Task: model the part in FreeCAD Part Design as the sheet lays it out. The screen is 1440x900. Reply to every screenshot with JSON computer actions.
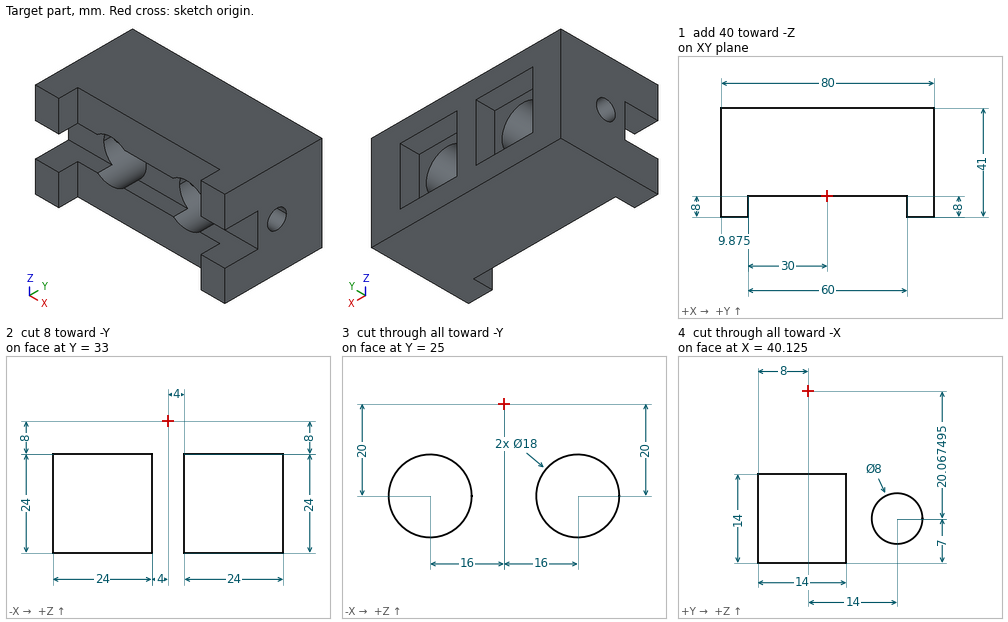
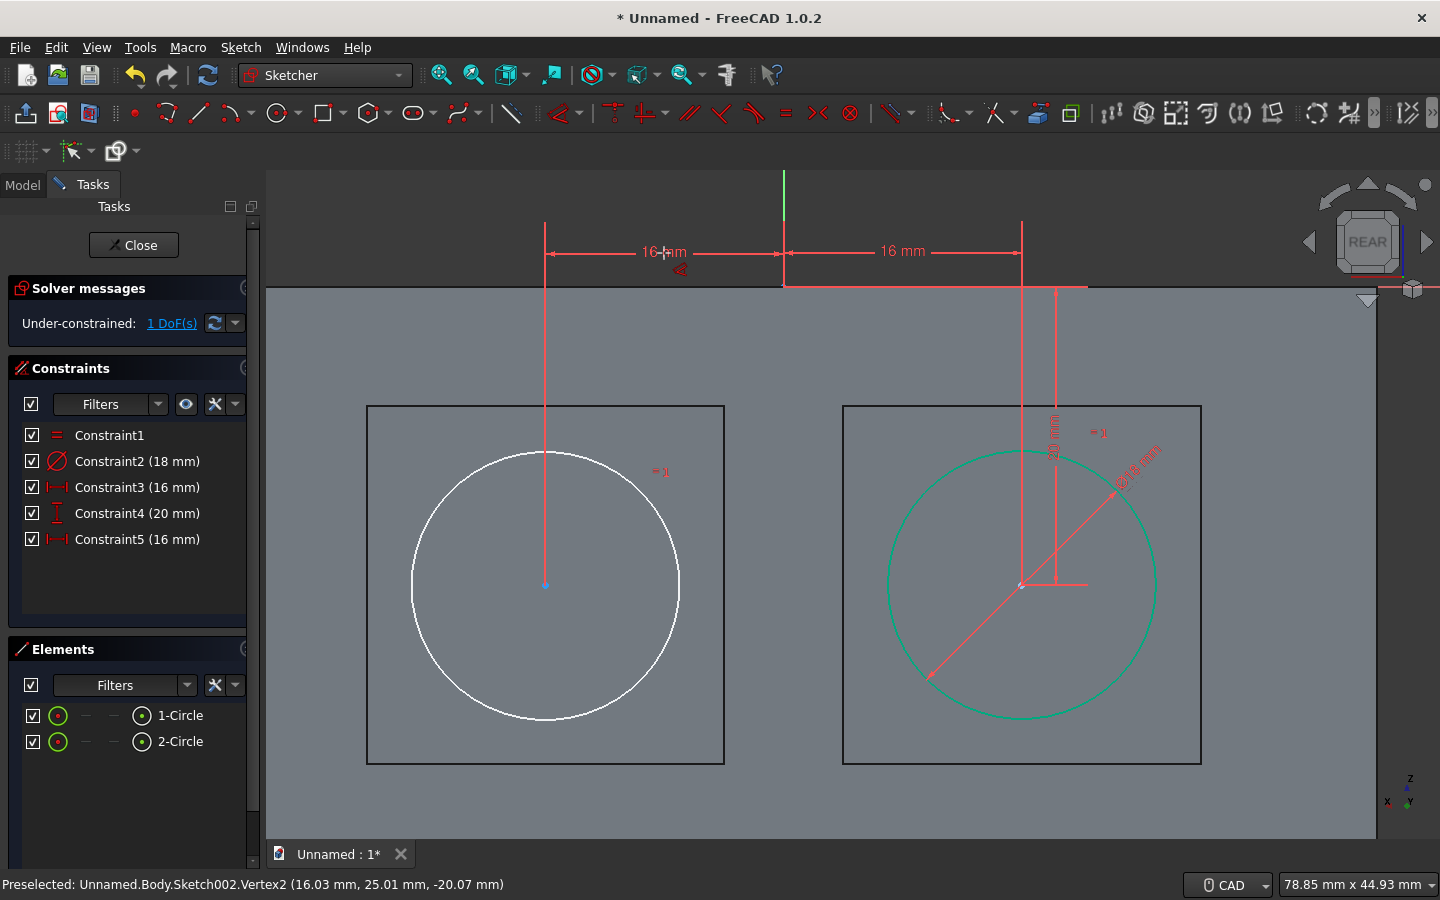
{"action": "left_click", "coordinate": [545, 586]}
{"action": "left_click", "coordinate": [511, 437]}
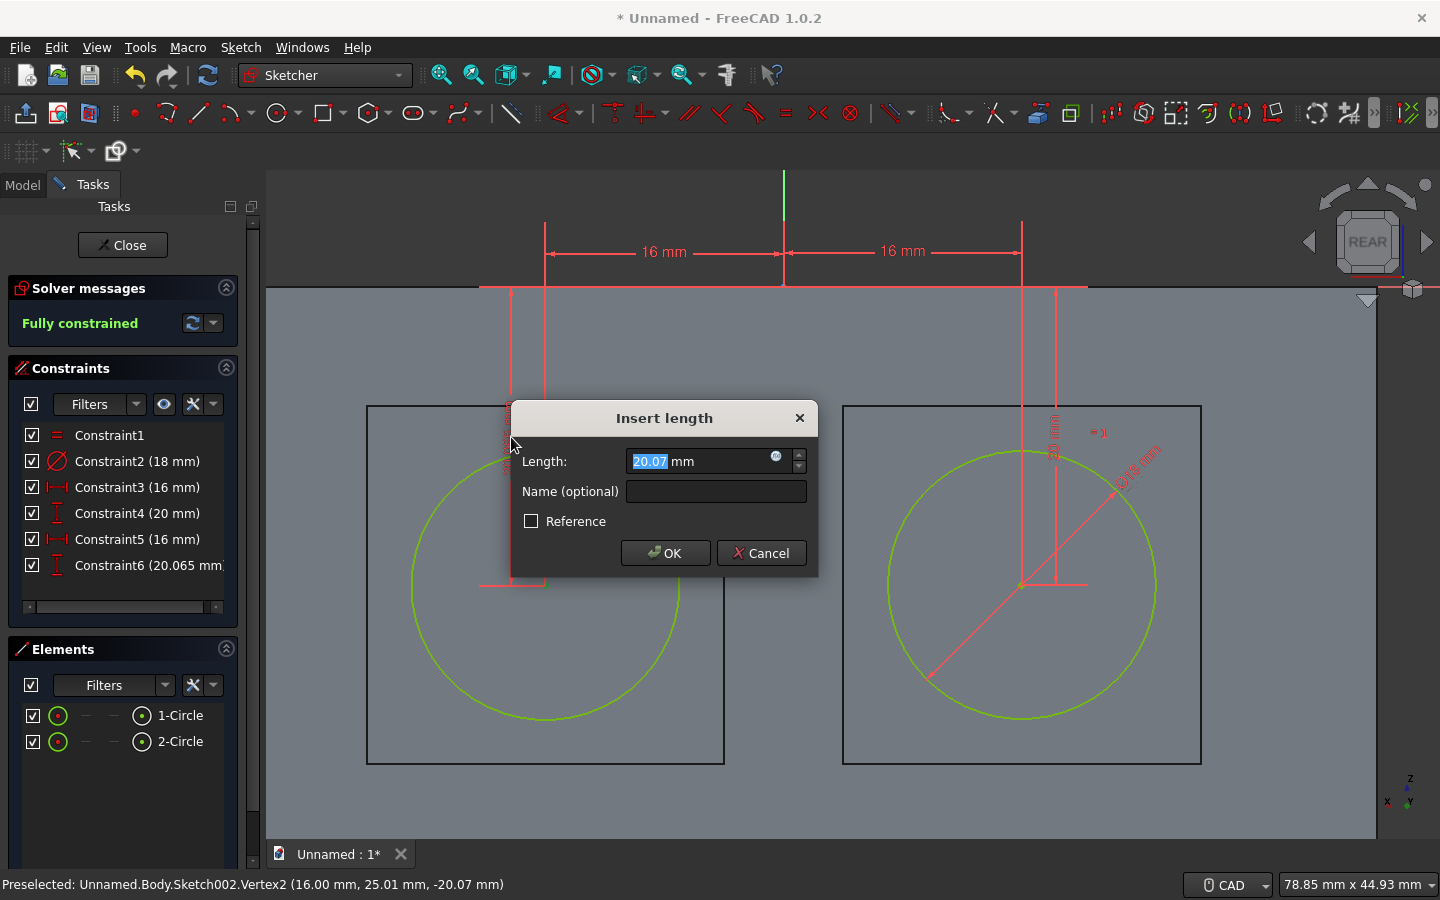
{"action": "type", "text": "20"}
{"action": "key", "text": "Return"}
{"action": "key", "text": "Escape"}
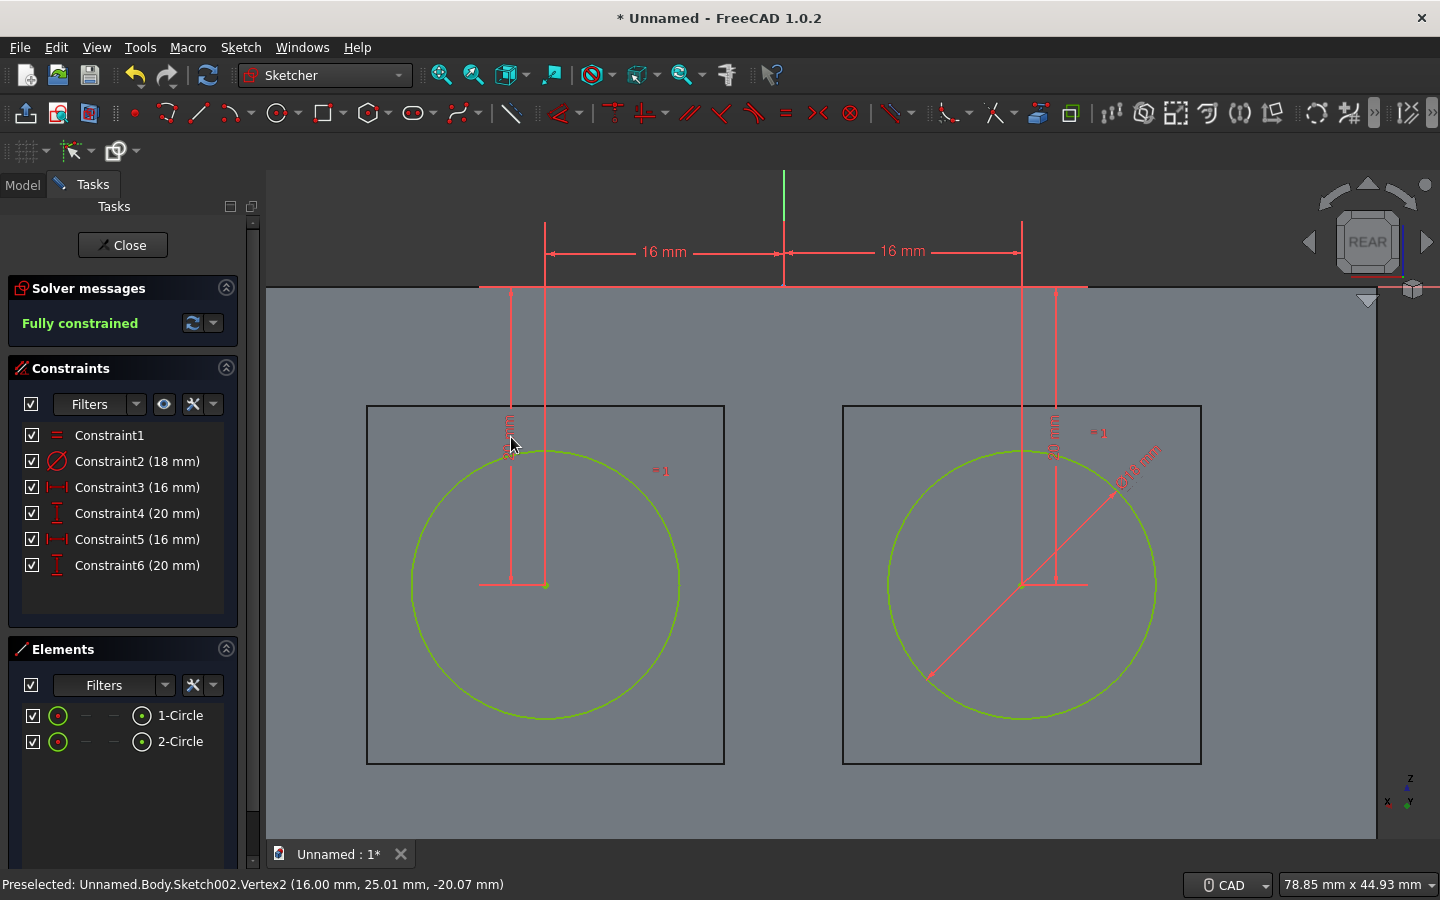
{"action": "left_click", "coordinate": [123, 245]}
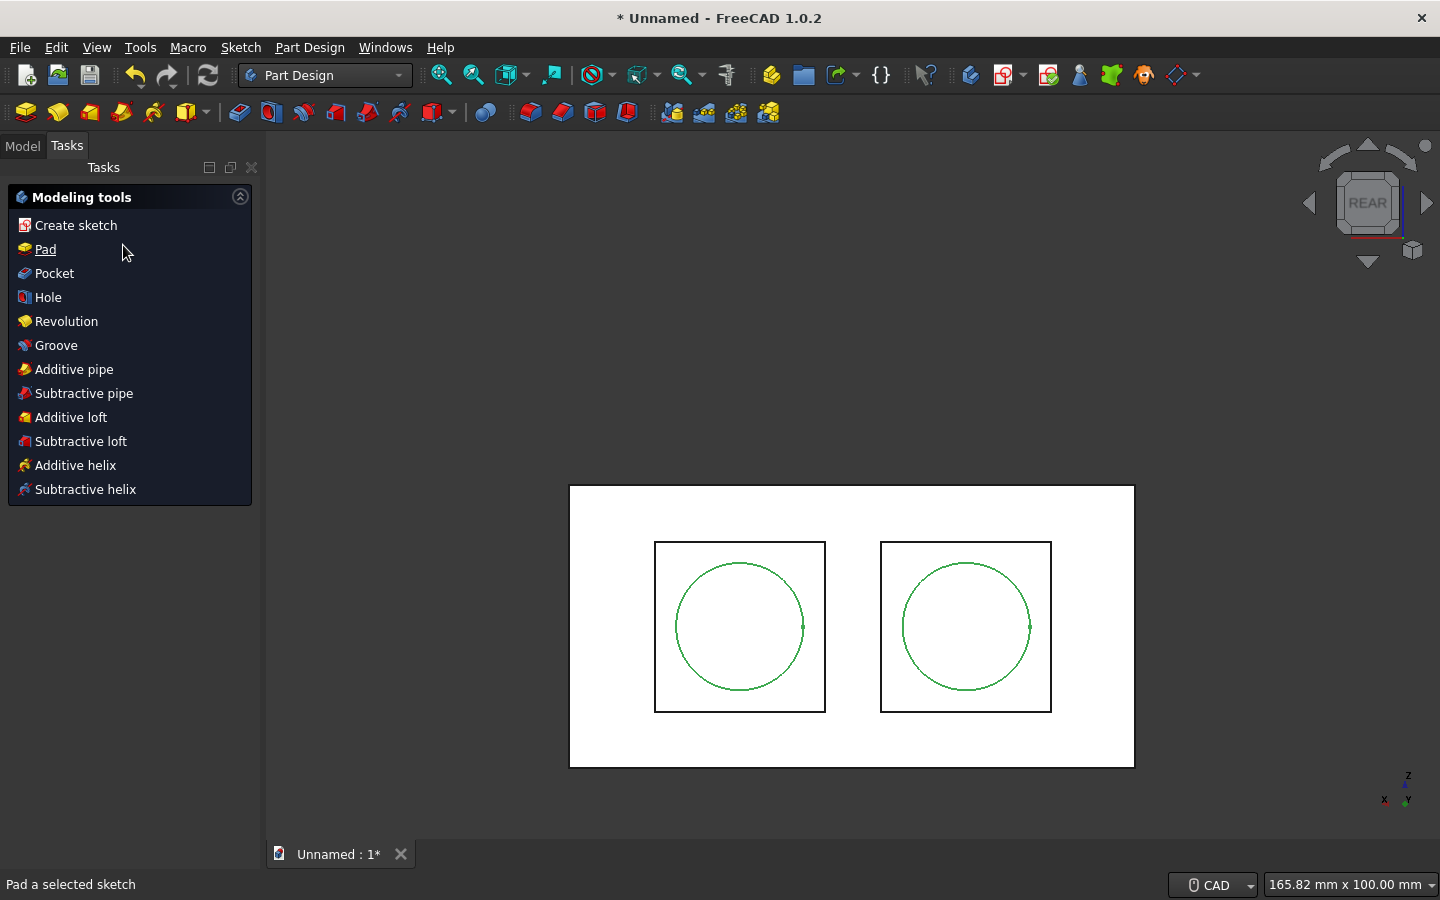
{"action": "left_click", "coordinate": [240, 112]}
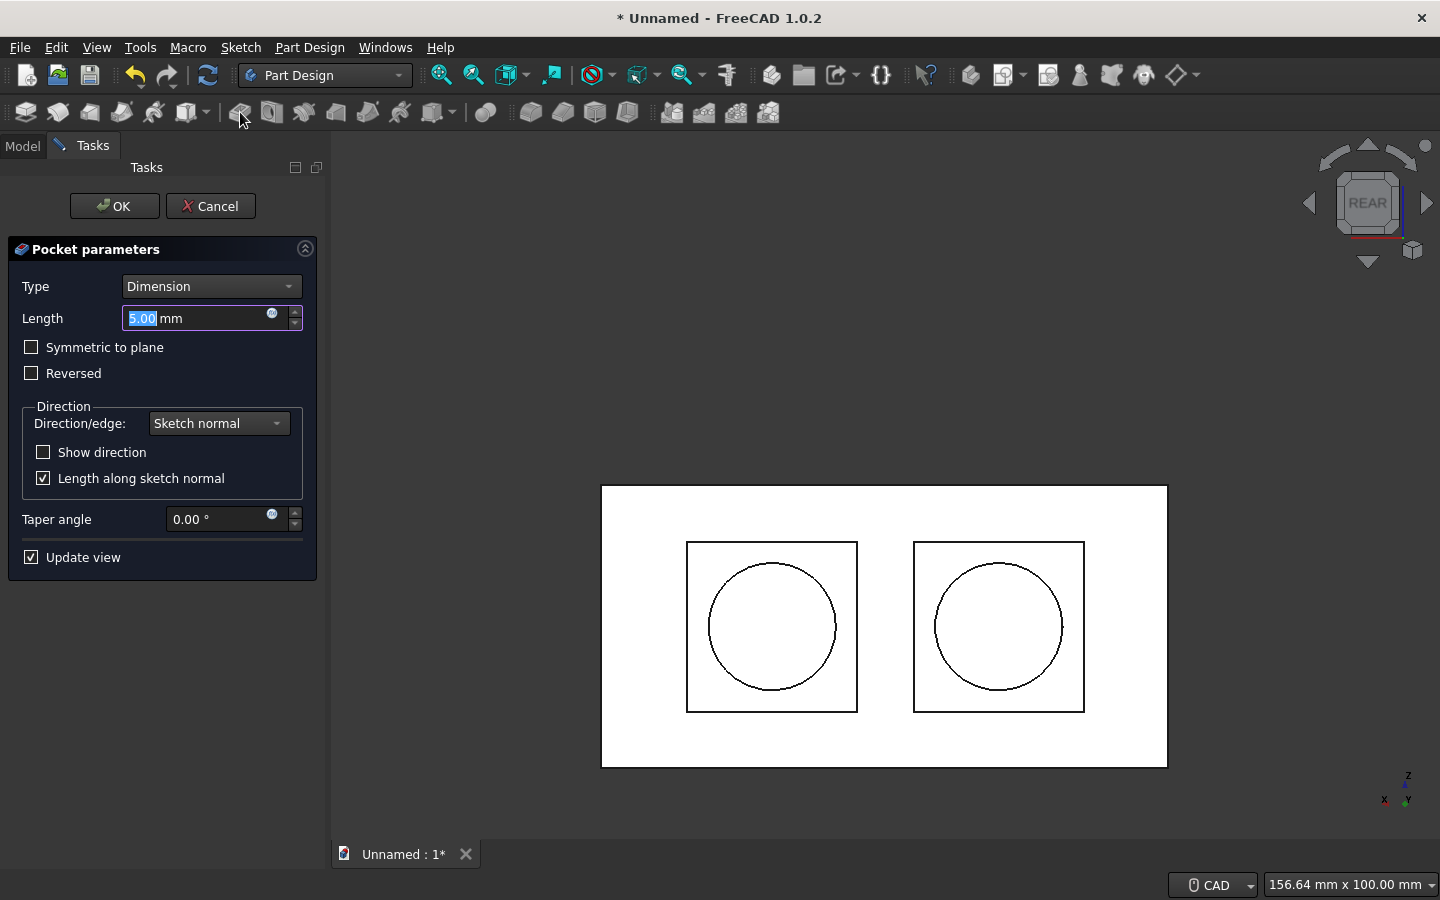
{"action": "left_click", "coordinate": [212, 286]}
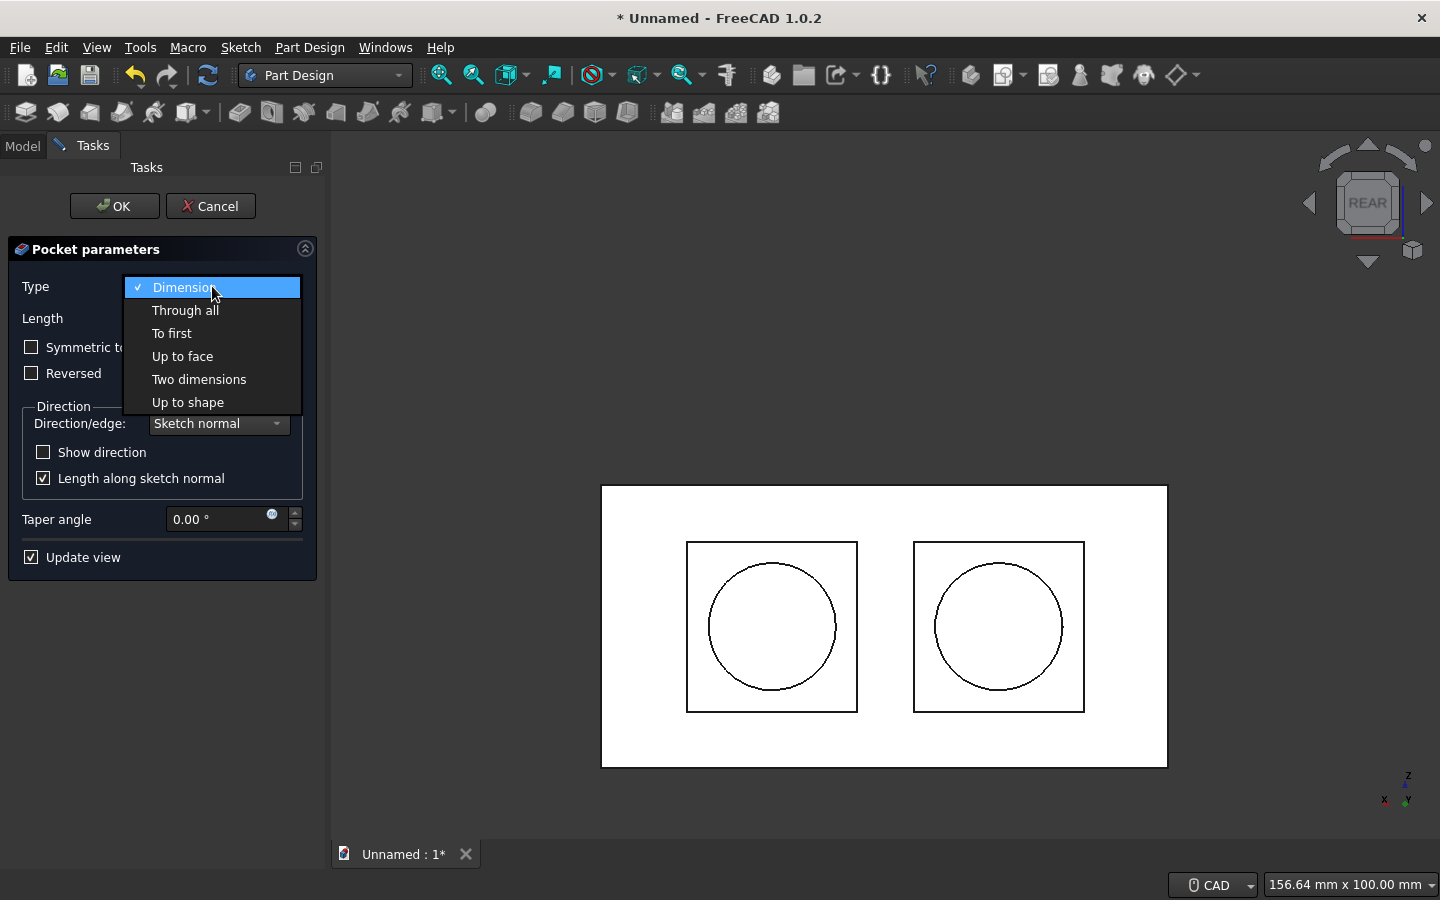
{"action": "left_click", "coordinate": [212, 310]}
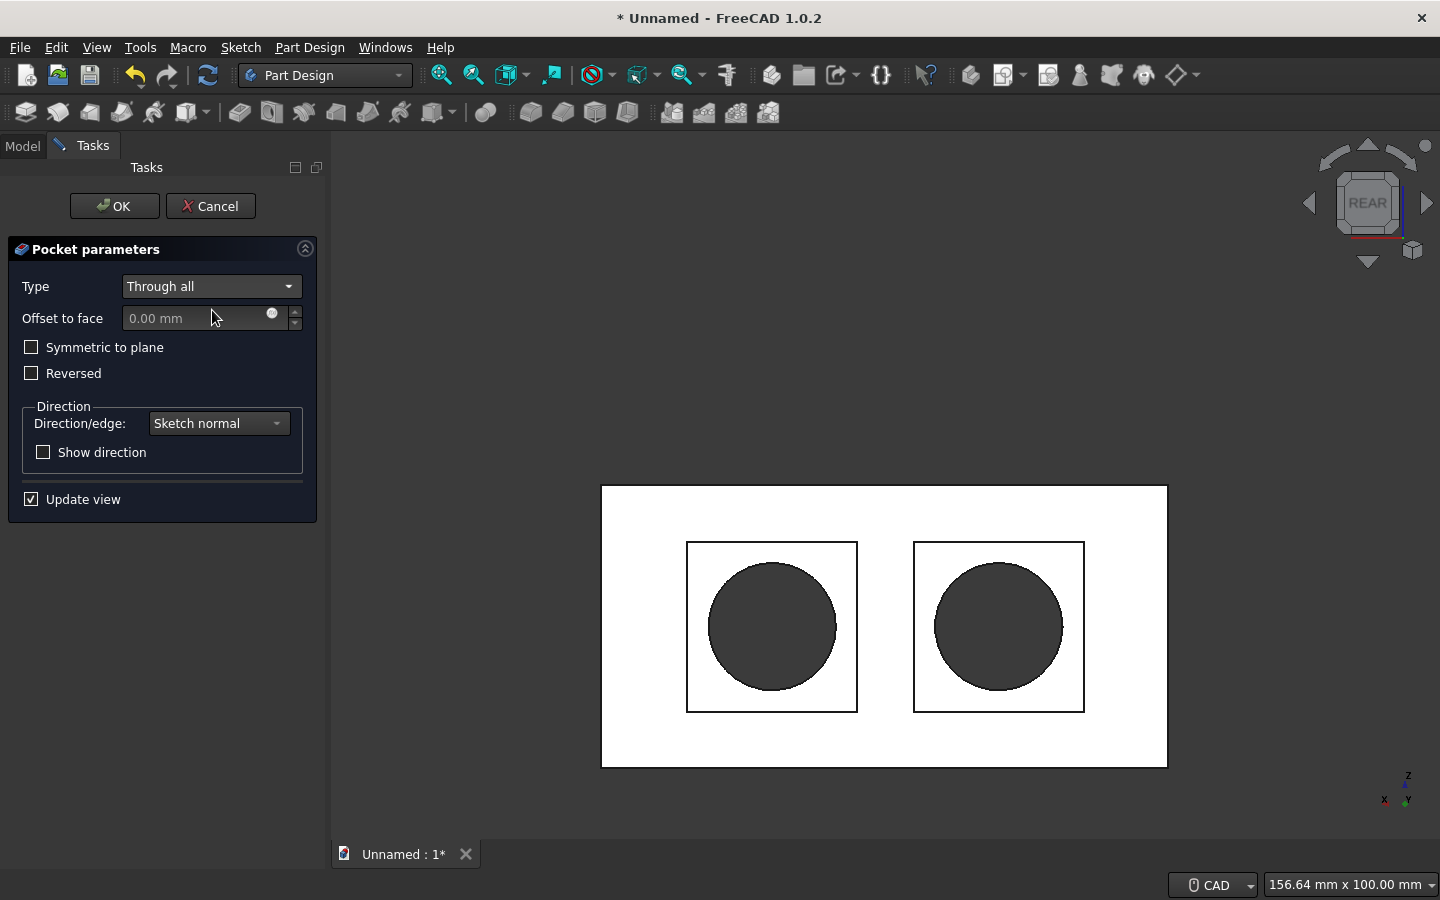
{"action": "left_click", "coordinate": [115, 206]}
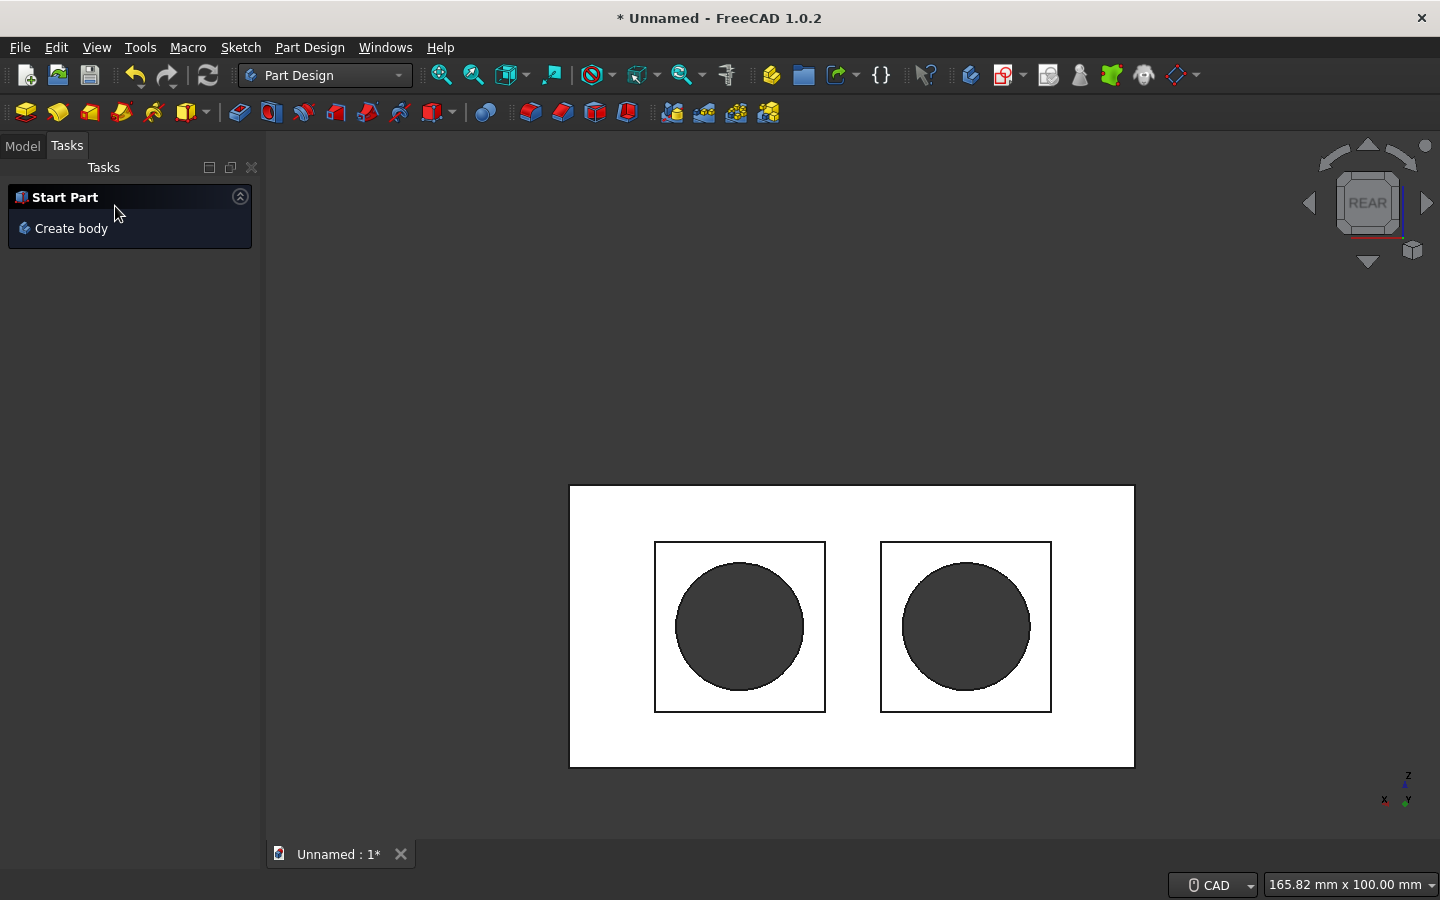
{"action": "key", "text": "0"}